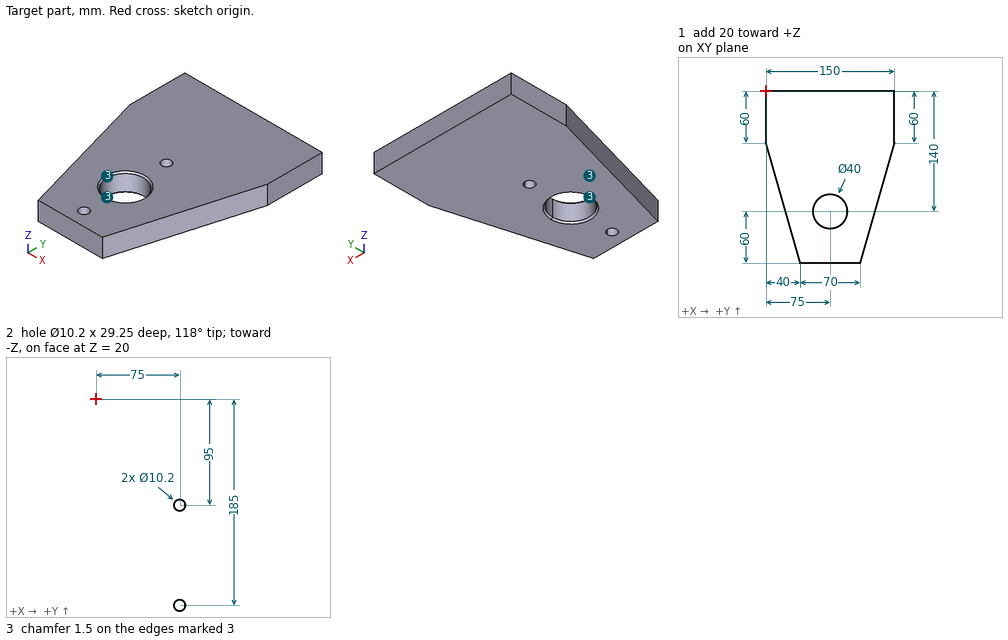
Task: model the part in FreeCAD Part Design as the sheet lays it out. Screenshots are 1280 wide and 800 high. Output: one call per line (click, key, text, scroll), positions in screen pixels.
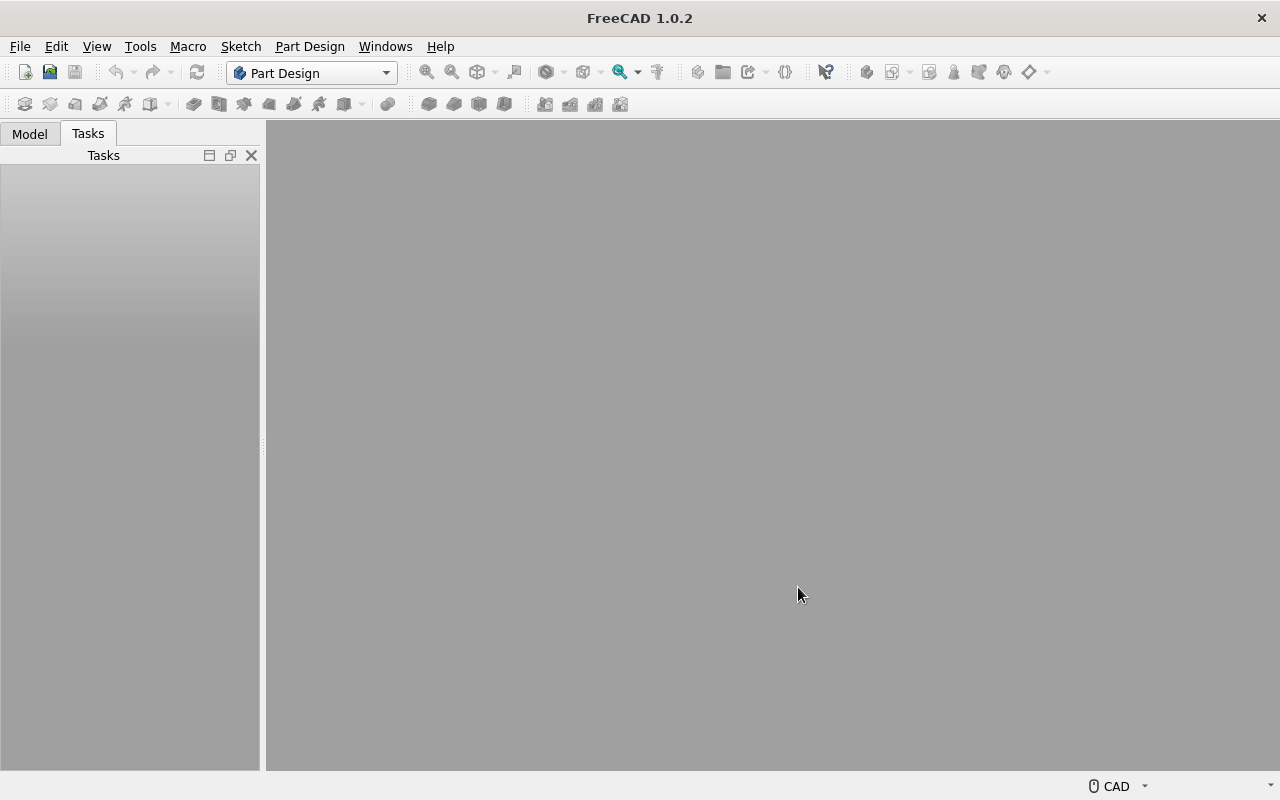
click(25, 72)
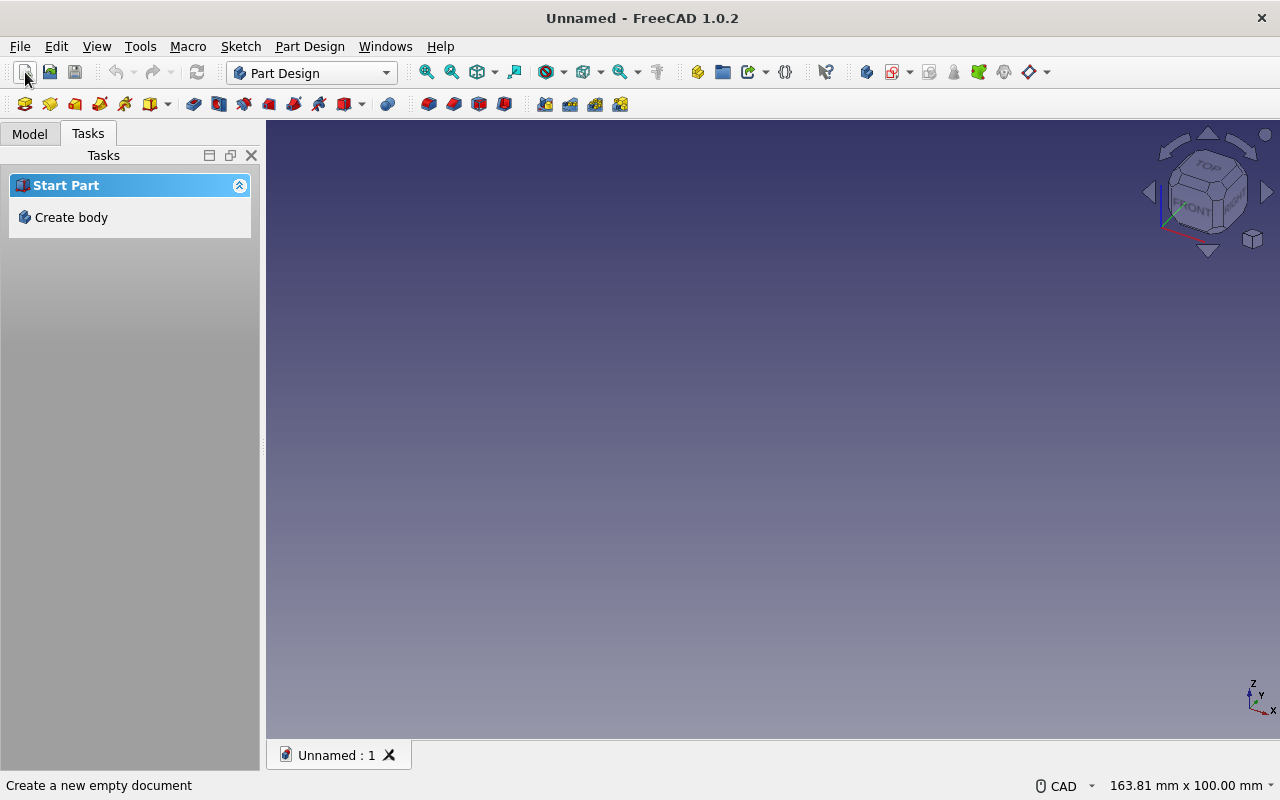
click(892, 72)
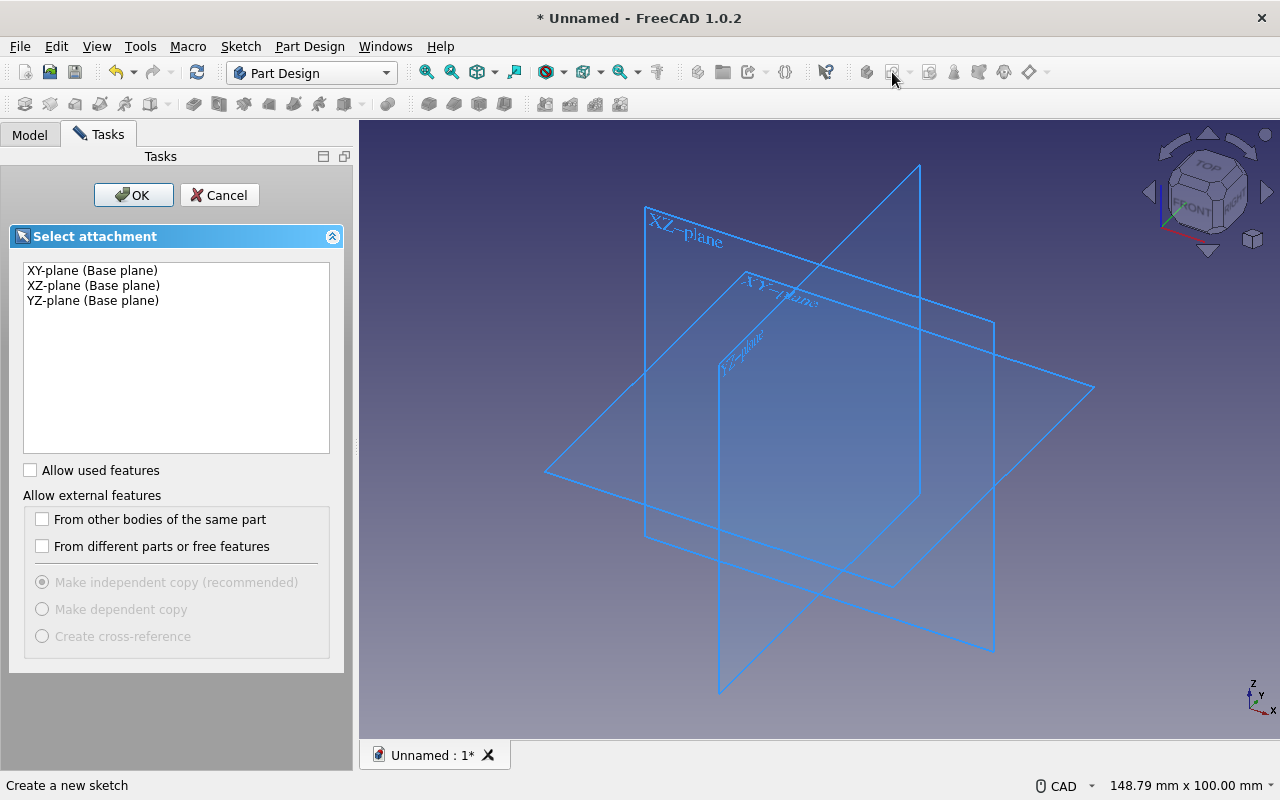
click(84, 270)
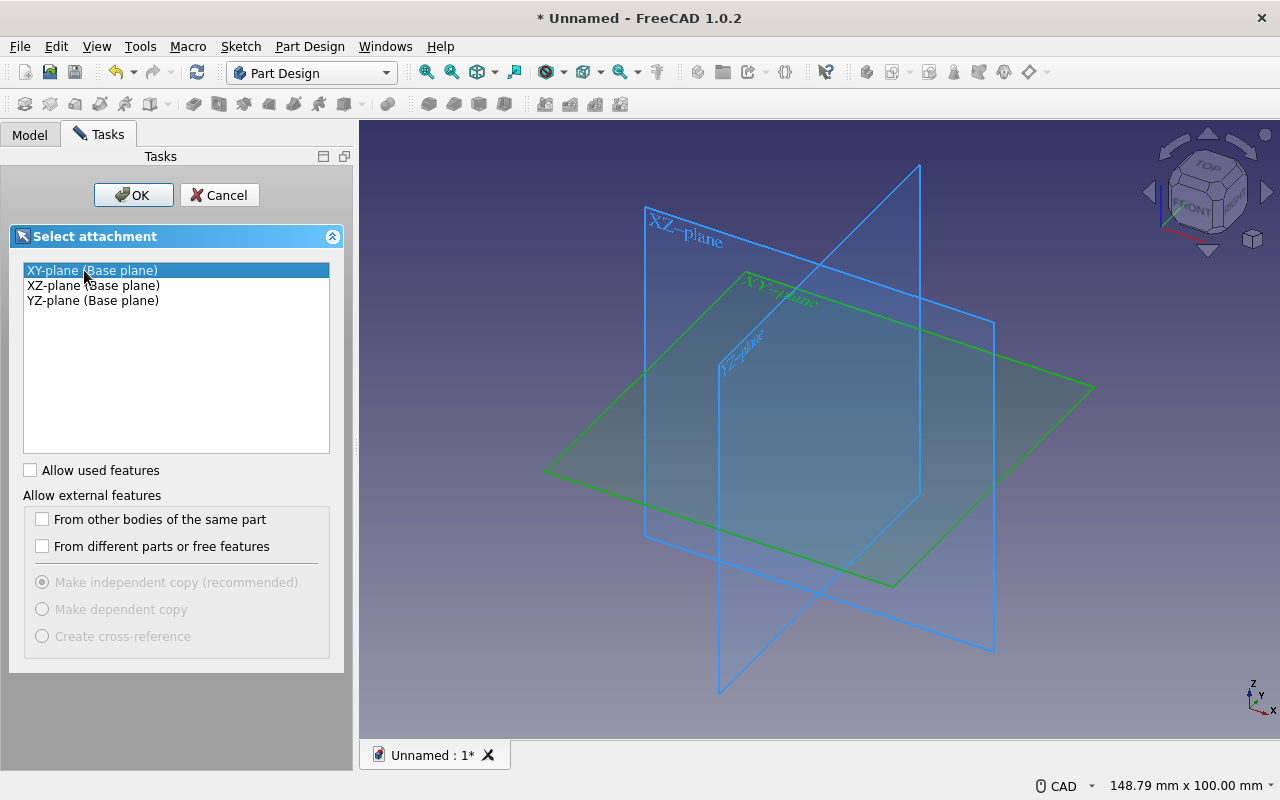
click(134, 195)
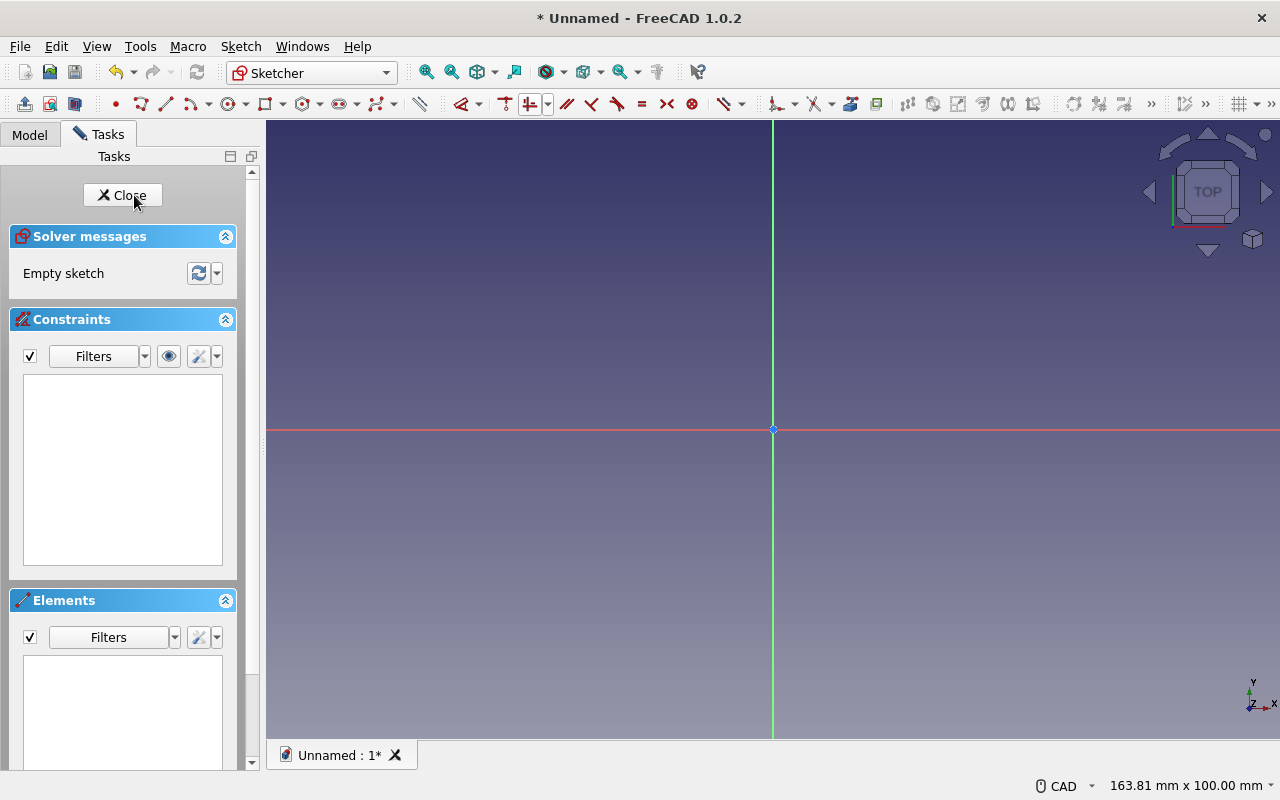
scroll(475, 163, down, 6)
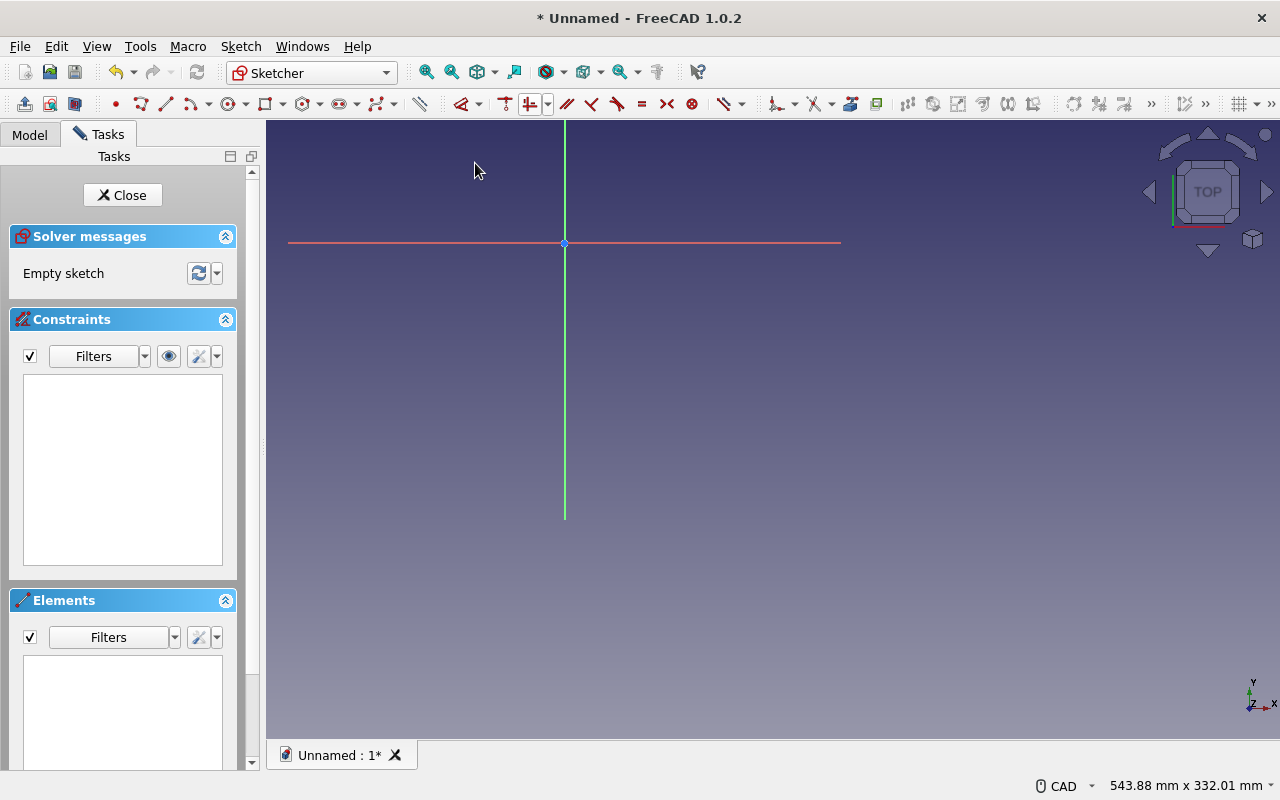
key(g)
key(m)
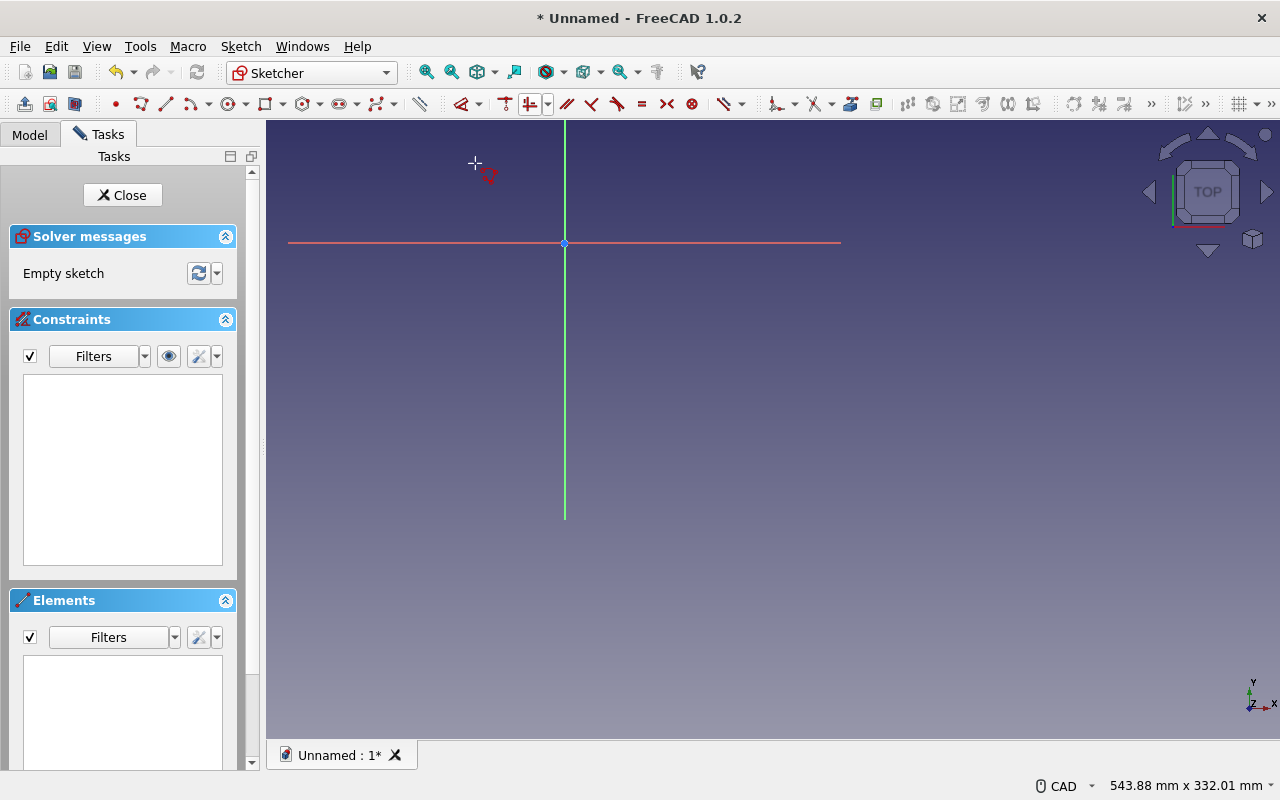
click(565, 243)
click(574, 355)
click(639, 616)
click(770, 616)
click(845, 355)
click(845, 252)
click(565, 243)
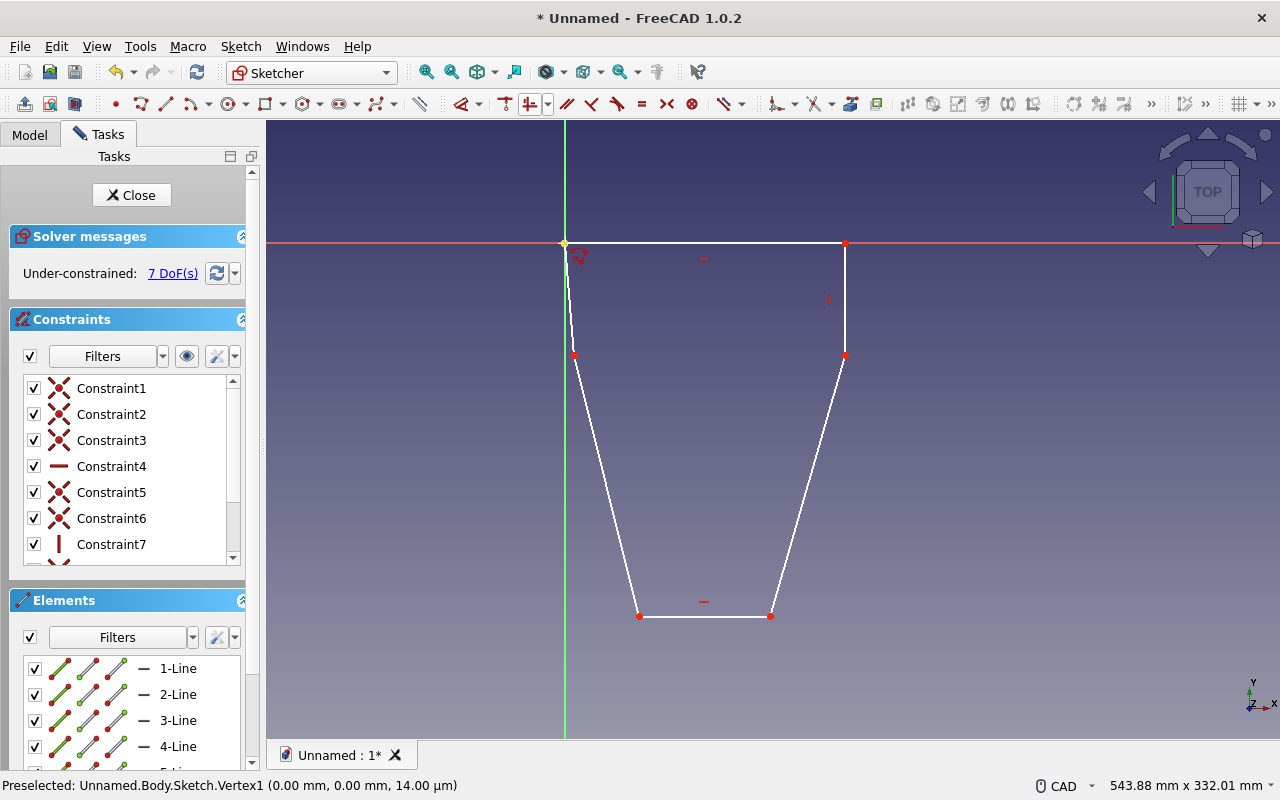
click(228, 104)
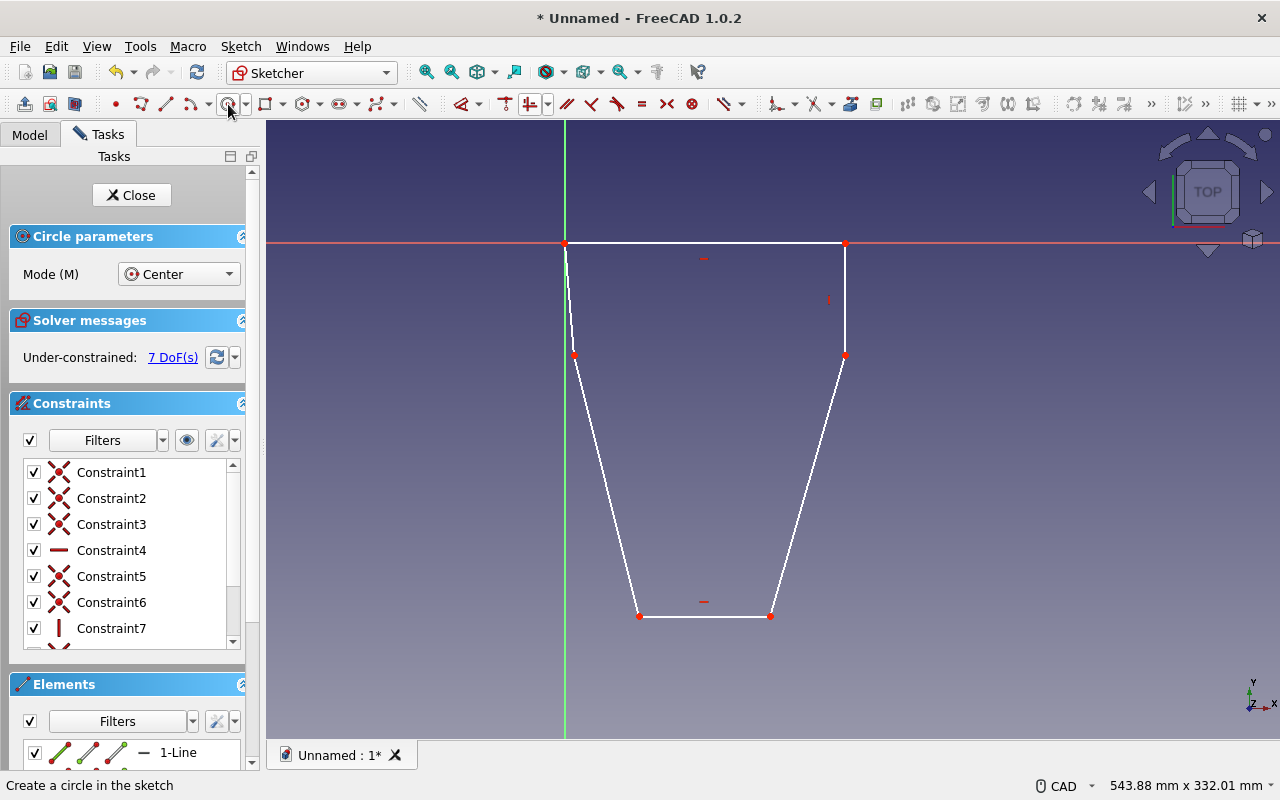
click(705, 504)
click(731, 478)
key(Escape)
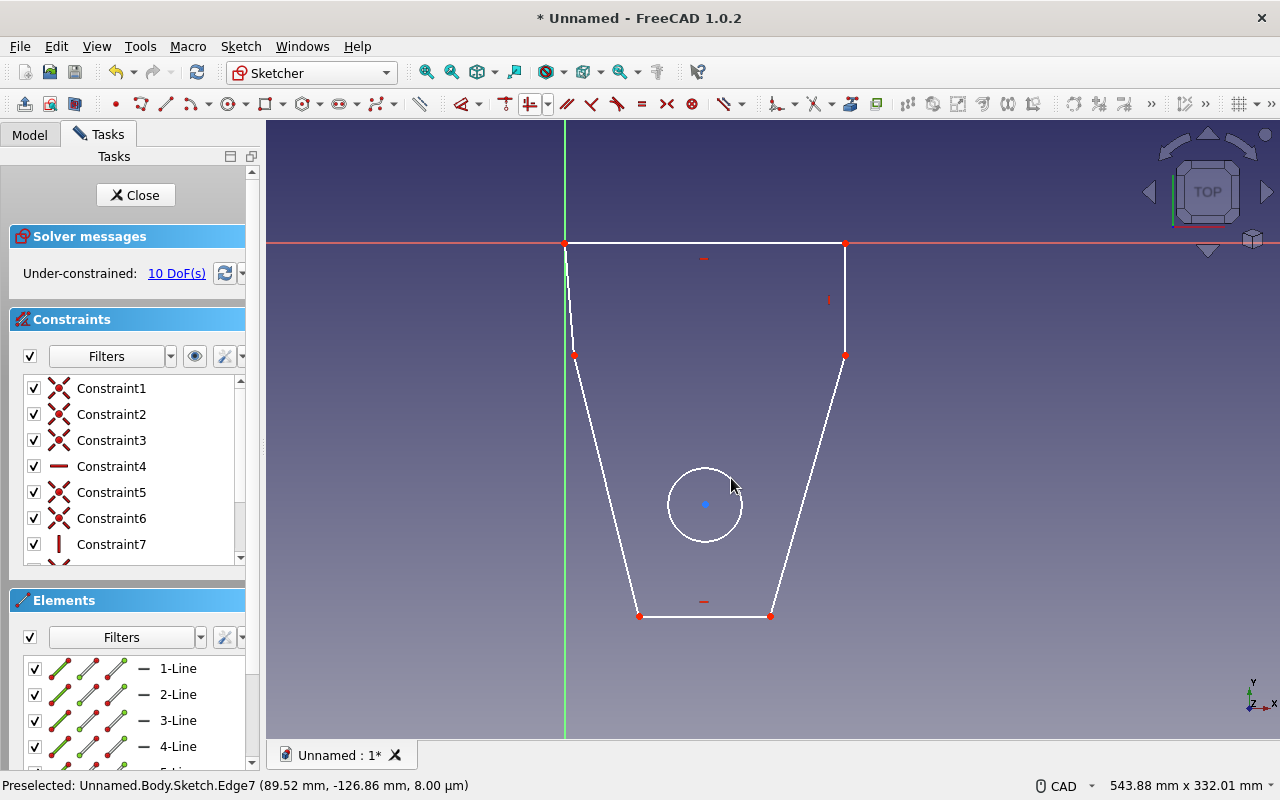
click(568, 277)